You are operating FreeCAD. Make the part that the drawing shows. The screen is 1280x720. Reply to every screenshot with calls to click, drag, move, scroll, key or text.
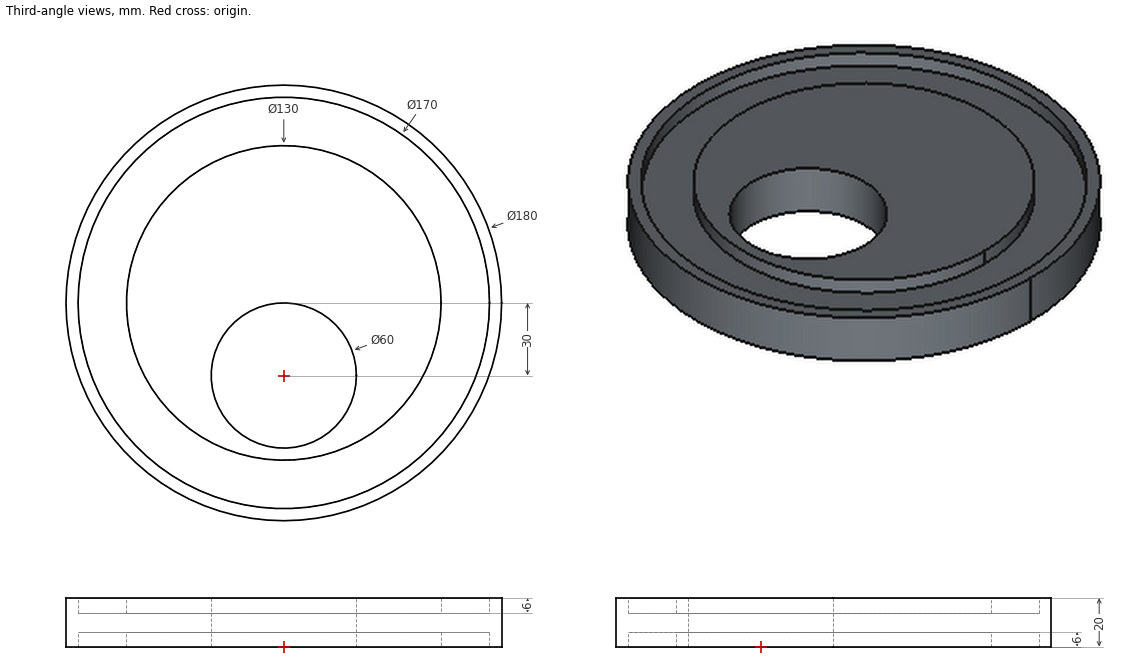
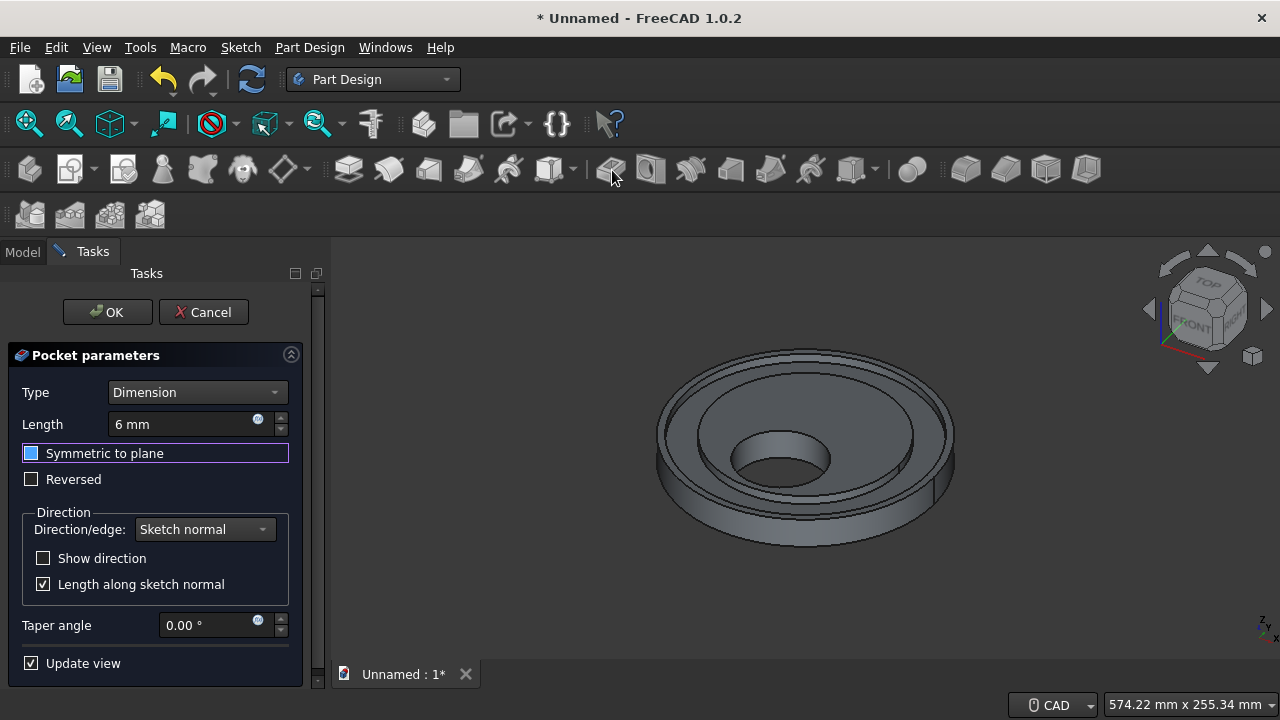
click(108, 312)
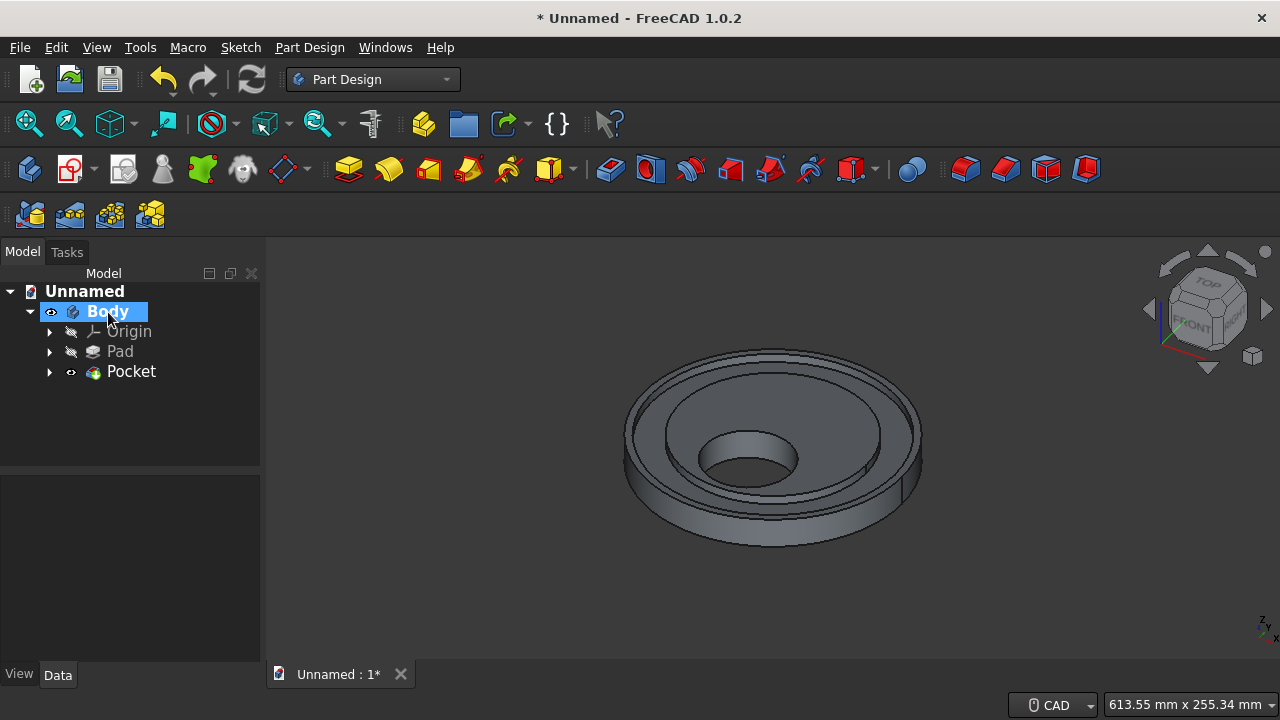
click(50, 332)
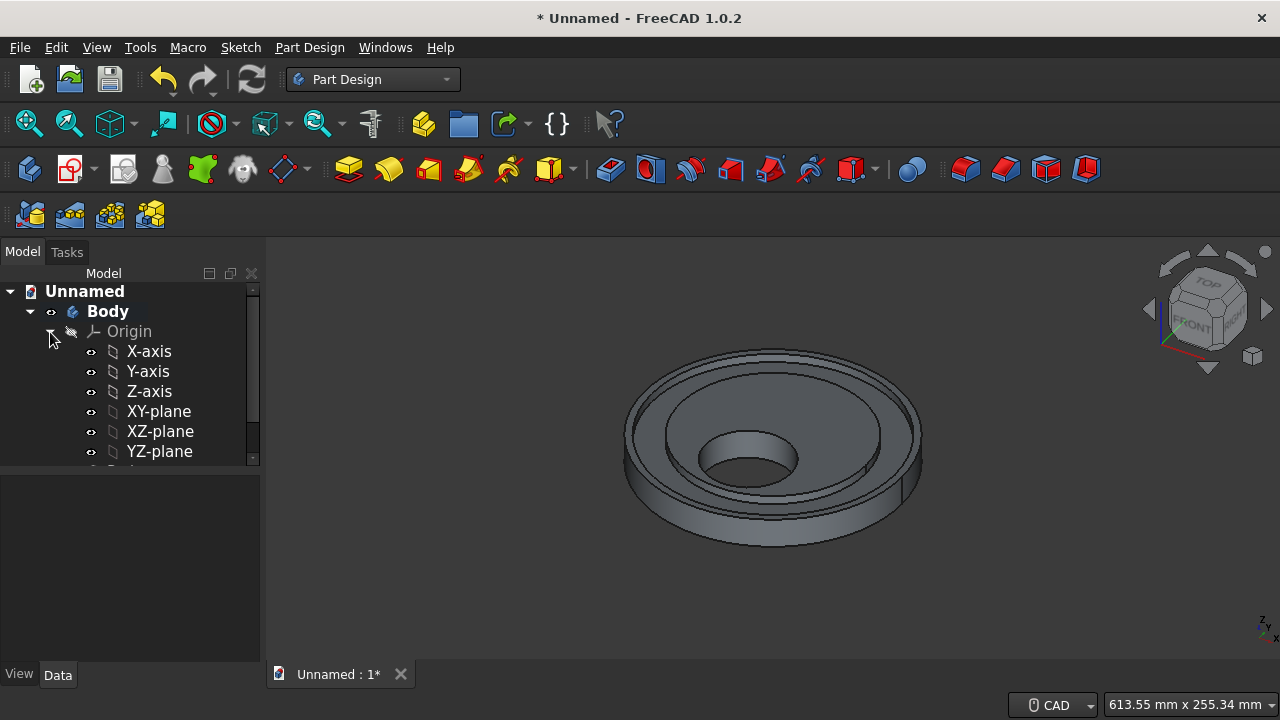
click(136, 412)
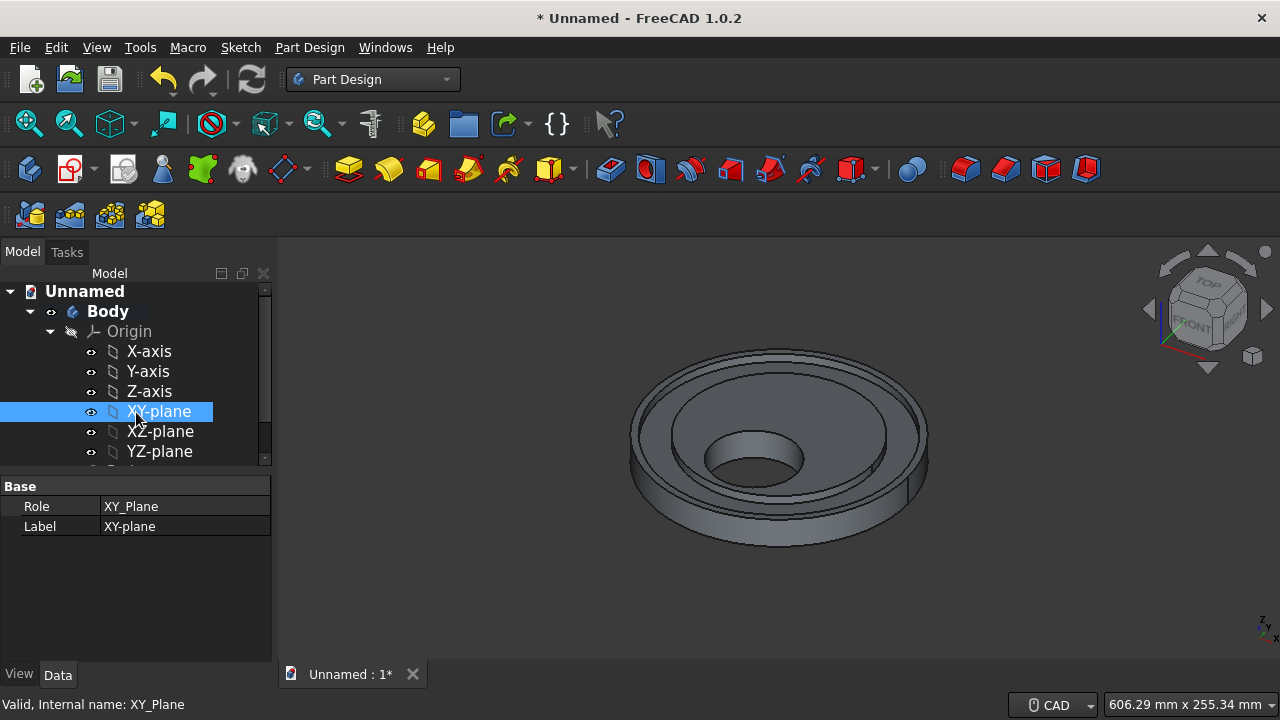
click(284, 170)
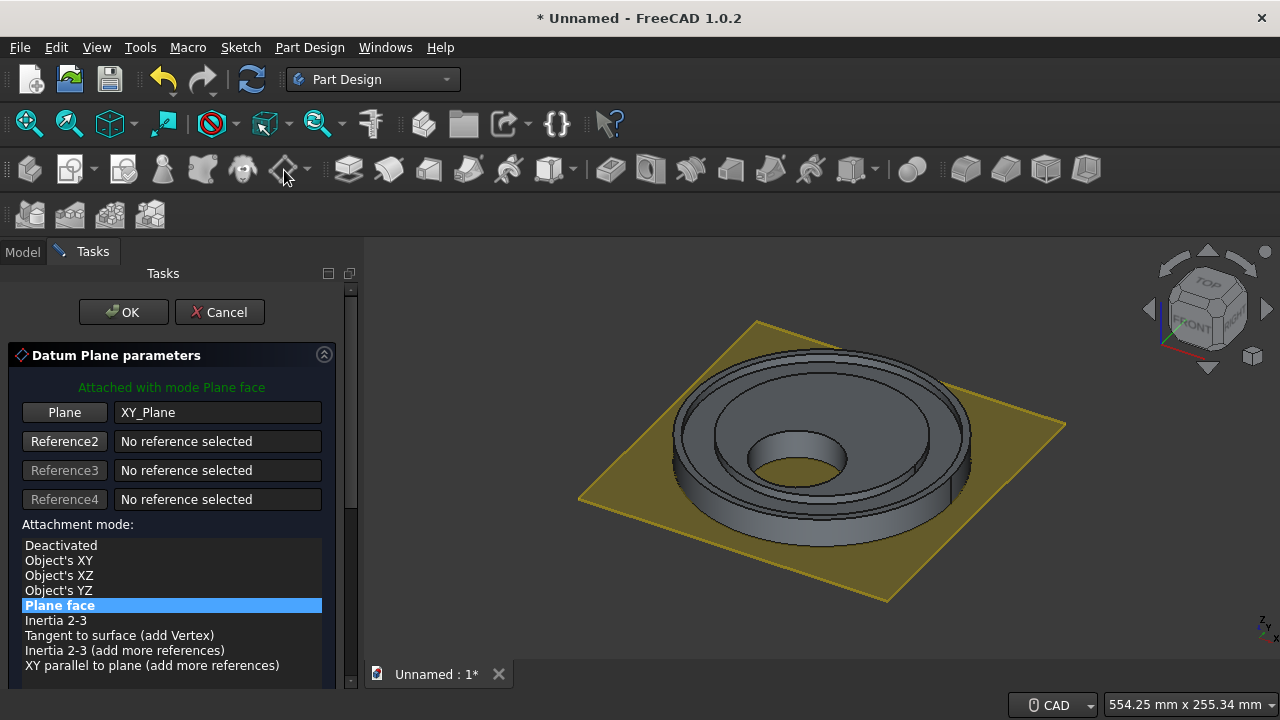
scroll(351, 486, down, 4)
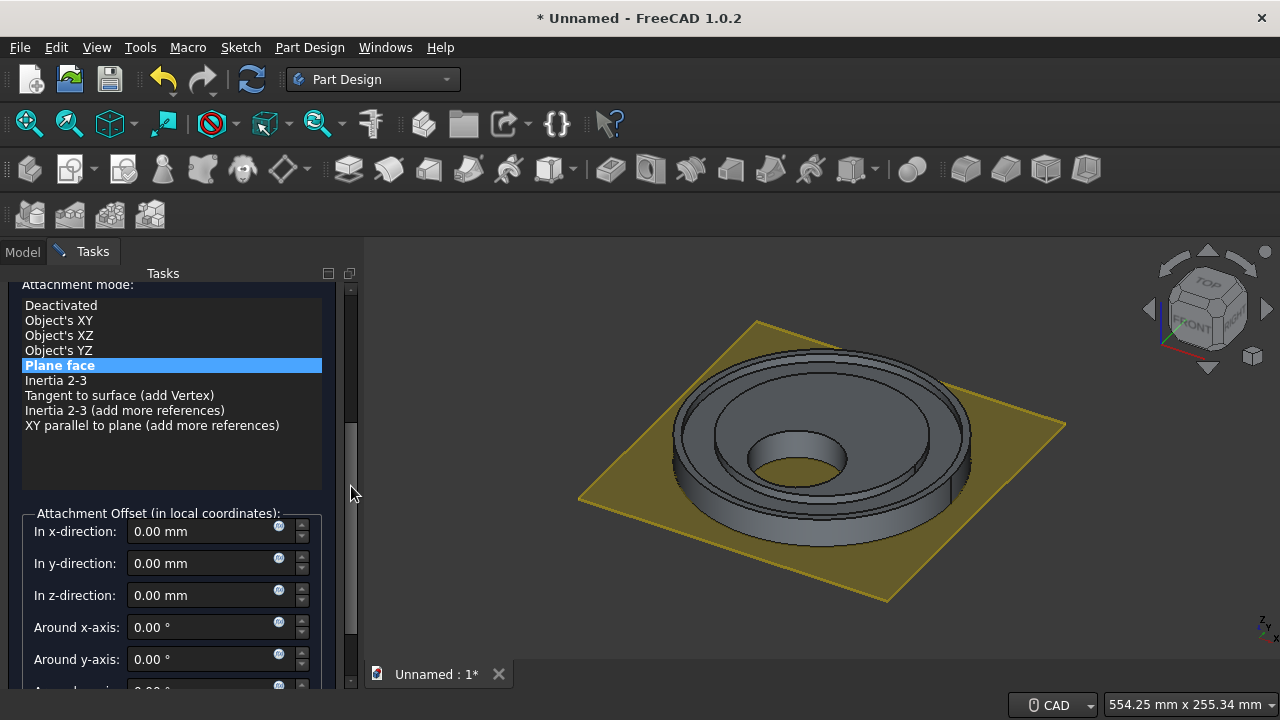
triple_click(210, 595)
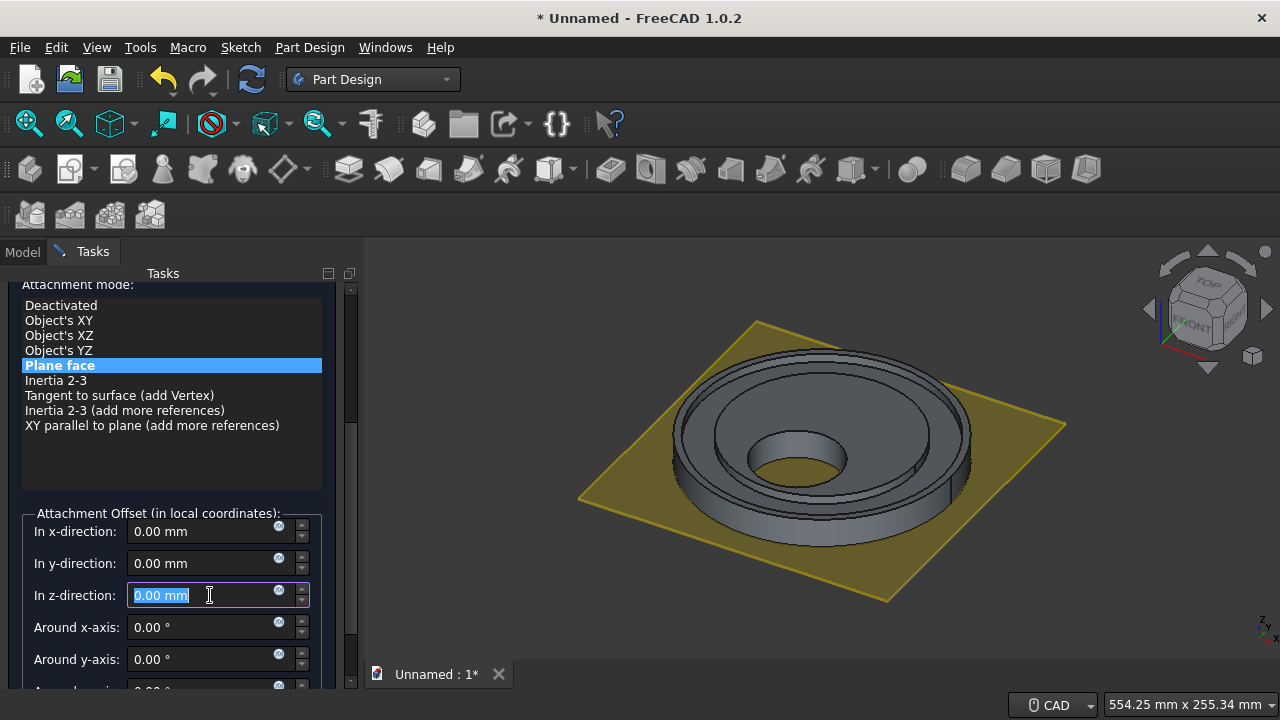
text(6)
key(Tab)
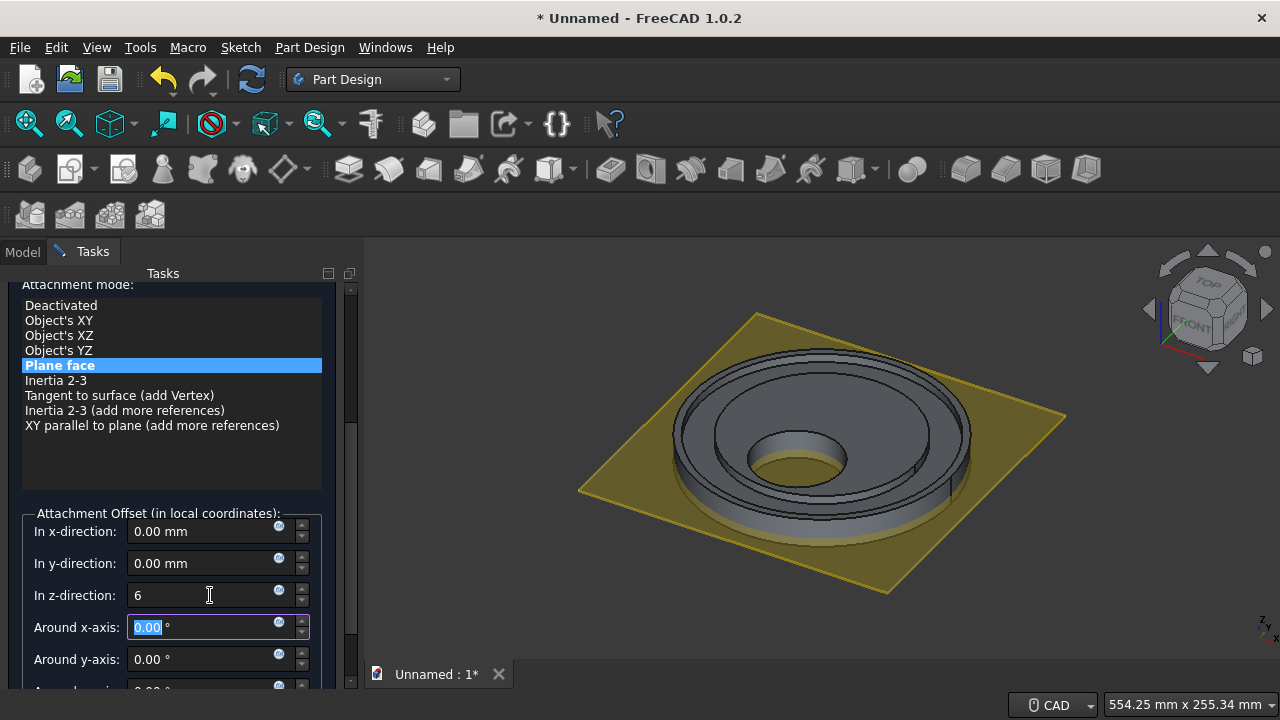
scroll(351, 486, up, 5)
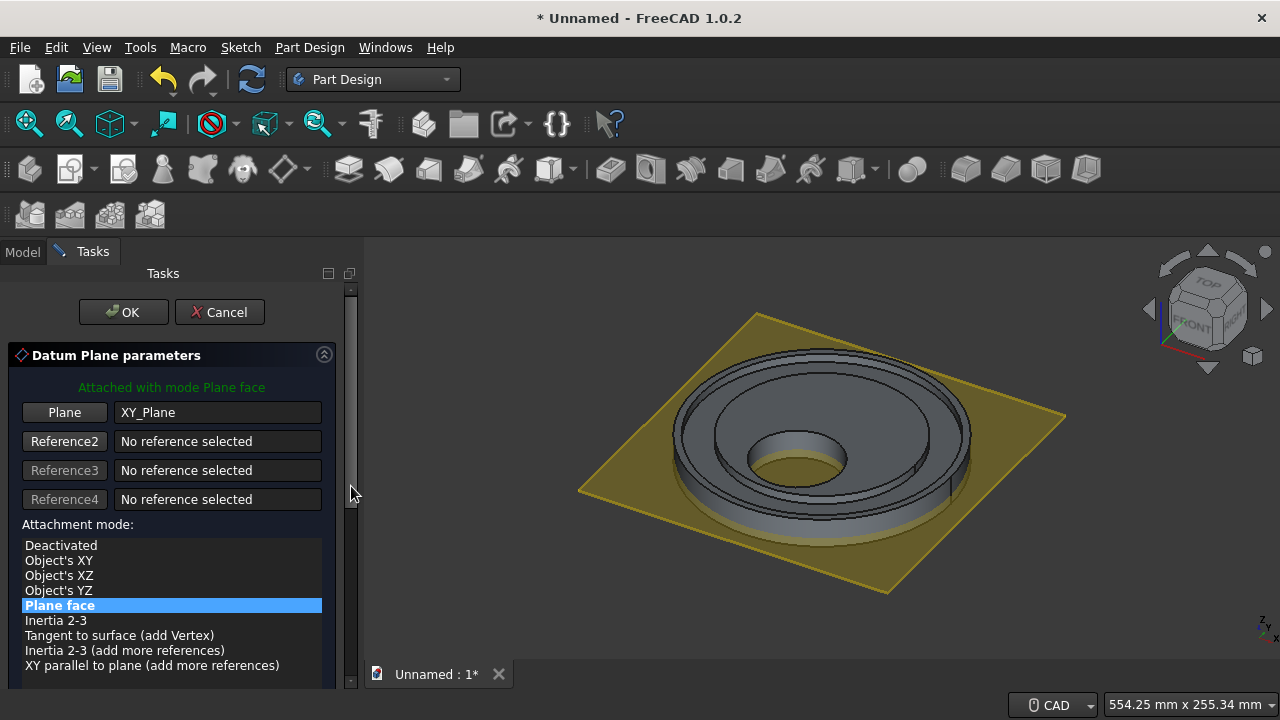
click(124, 312)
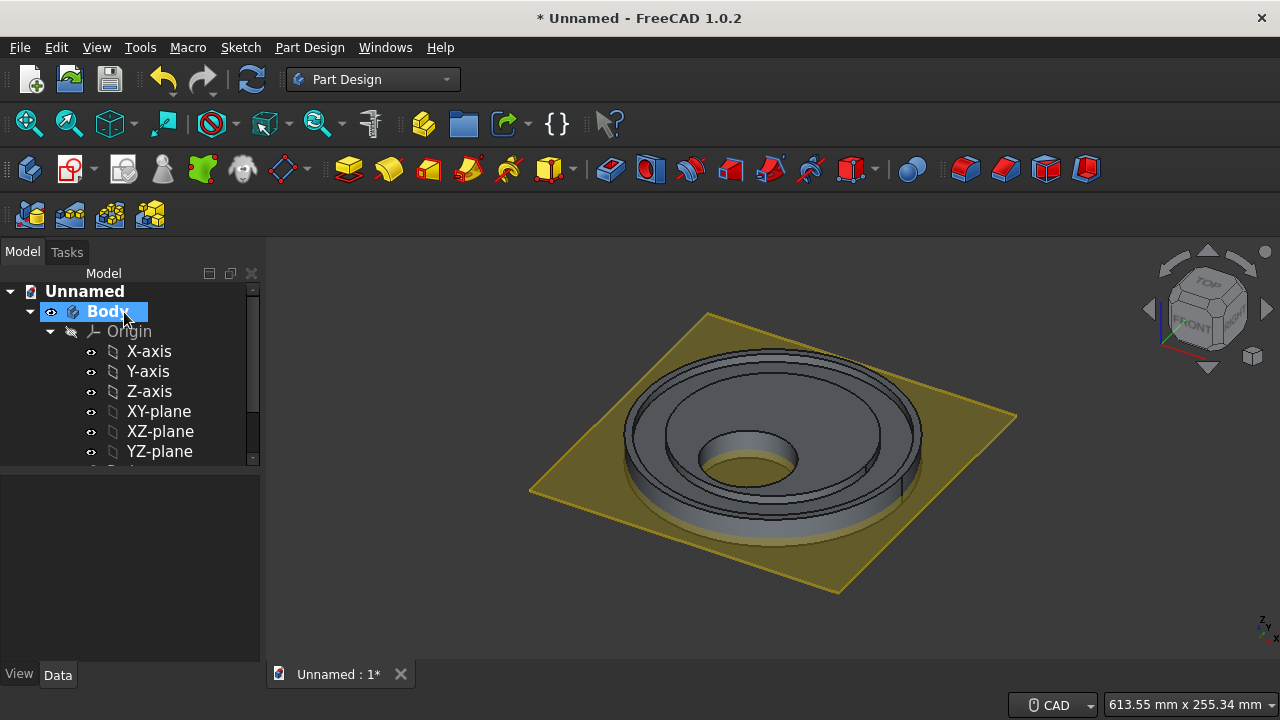
scroll(100, 367, down, 3)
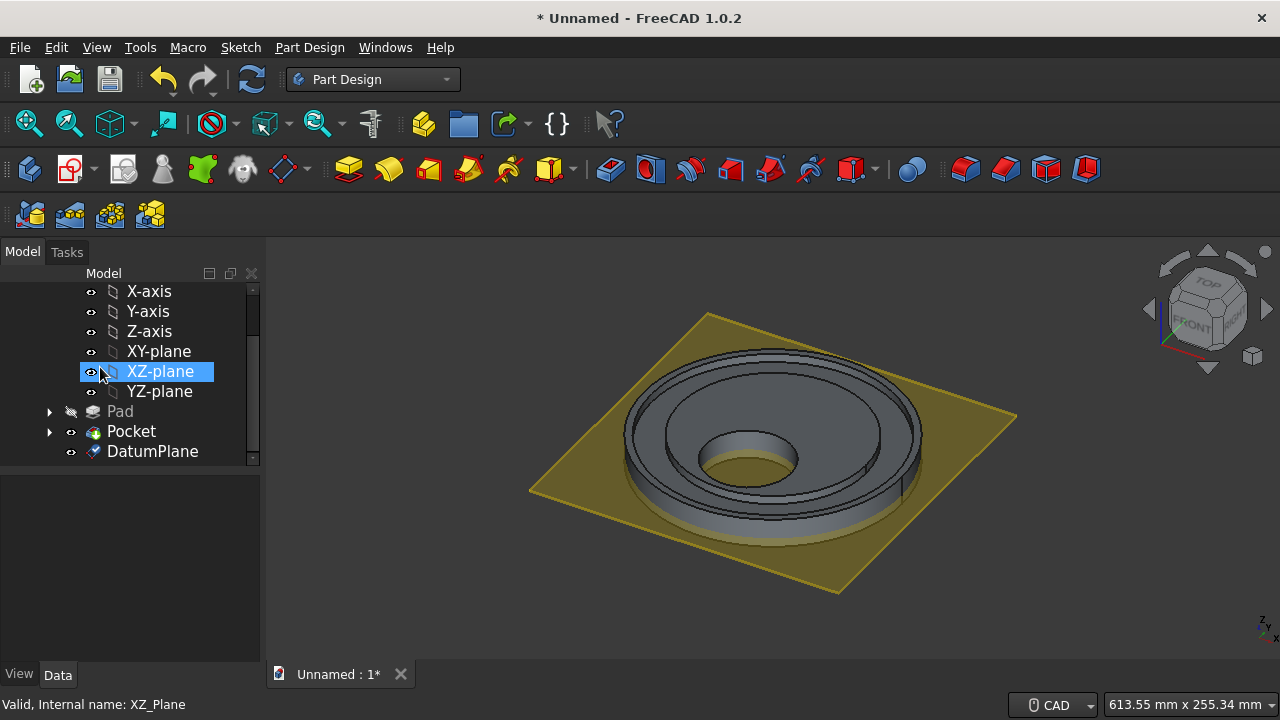
click(116, 452)